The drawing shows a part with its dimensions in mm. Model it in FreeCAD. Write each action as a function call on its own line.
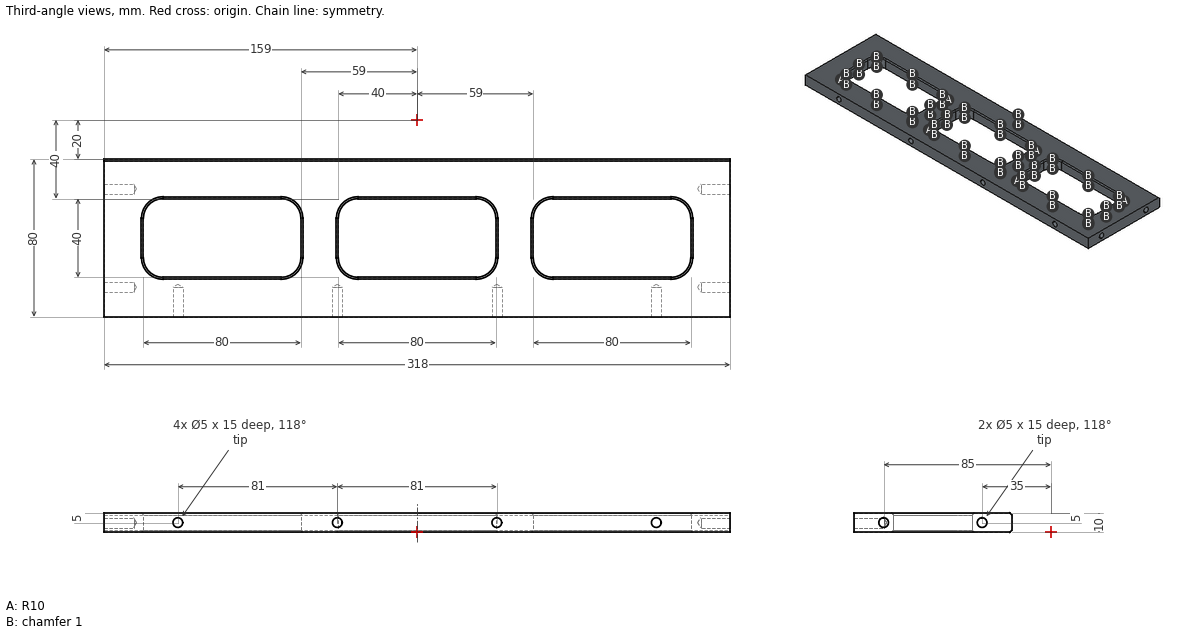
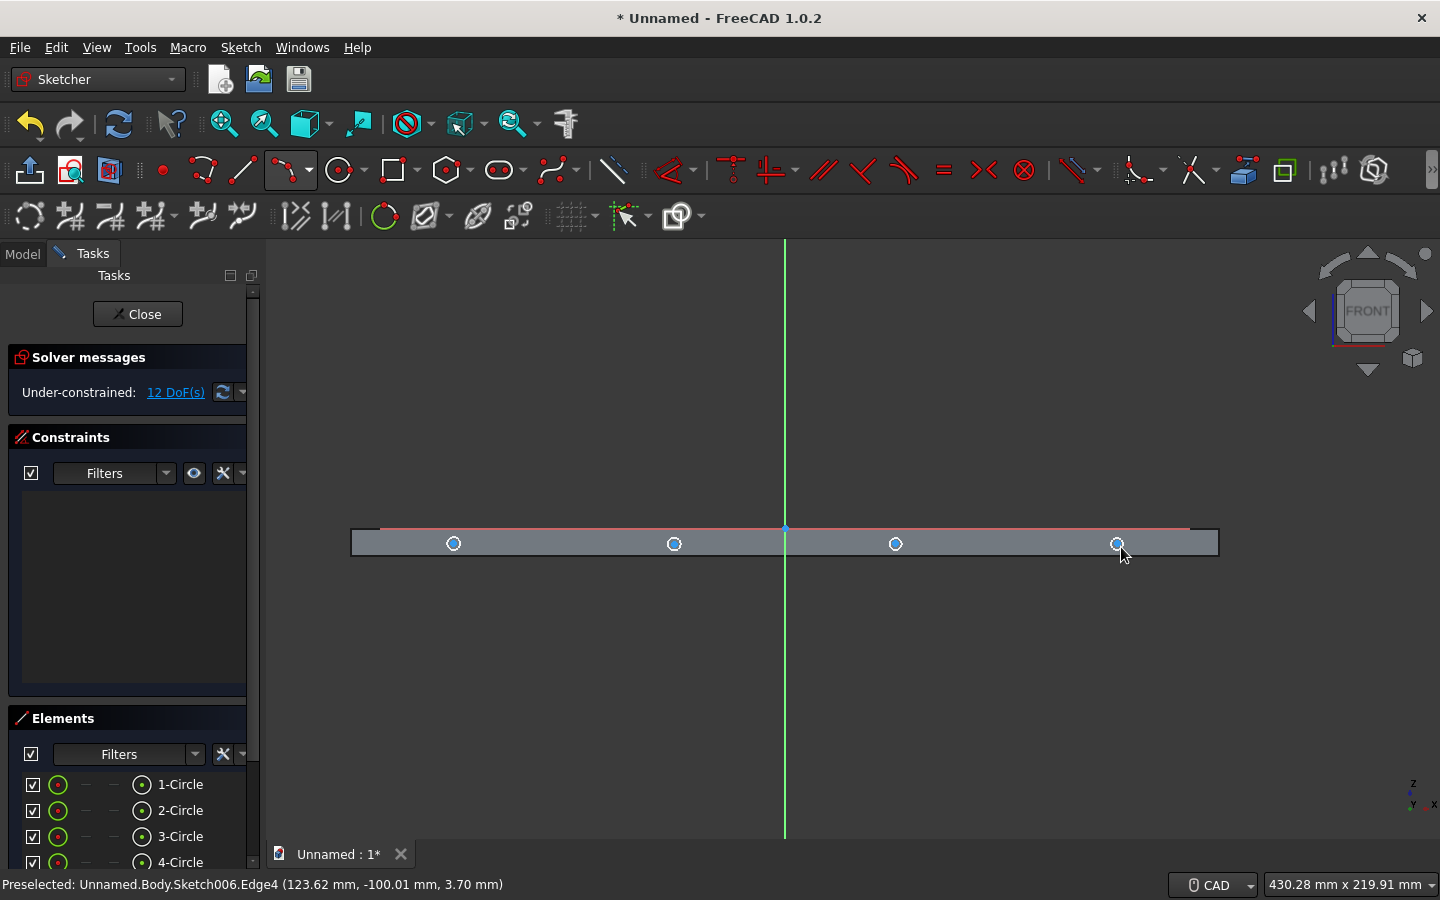
scroll(458, 539, up, 4)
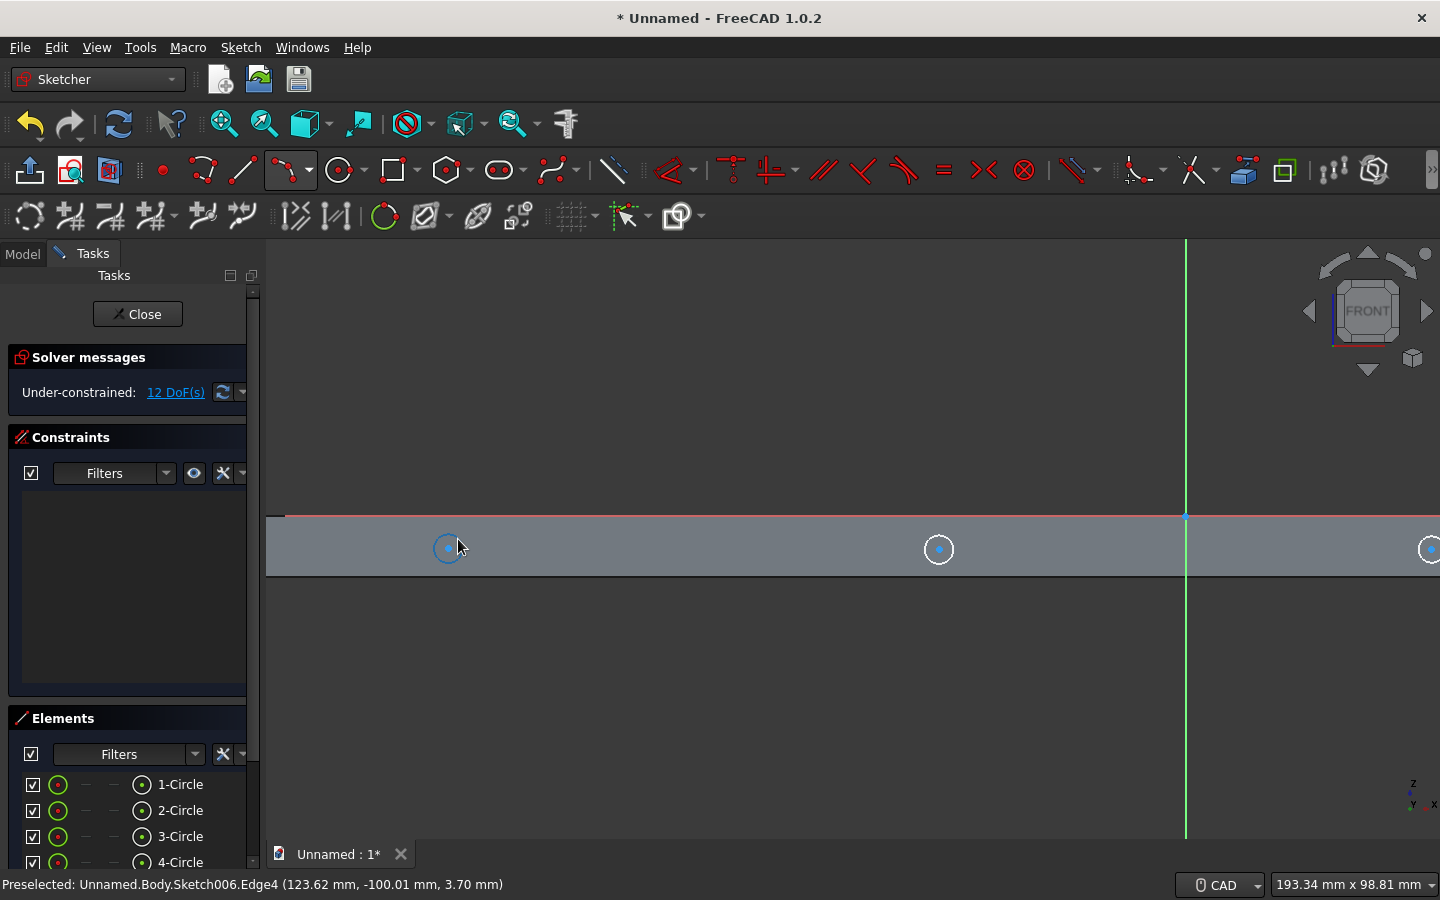
click(458, 539)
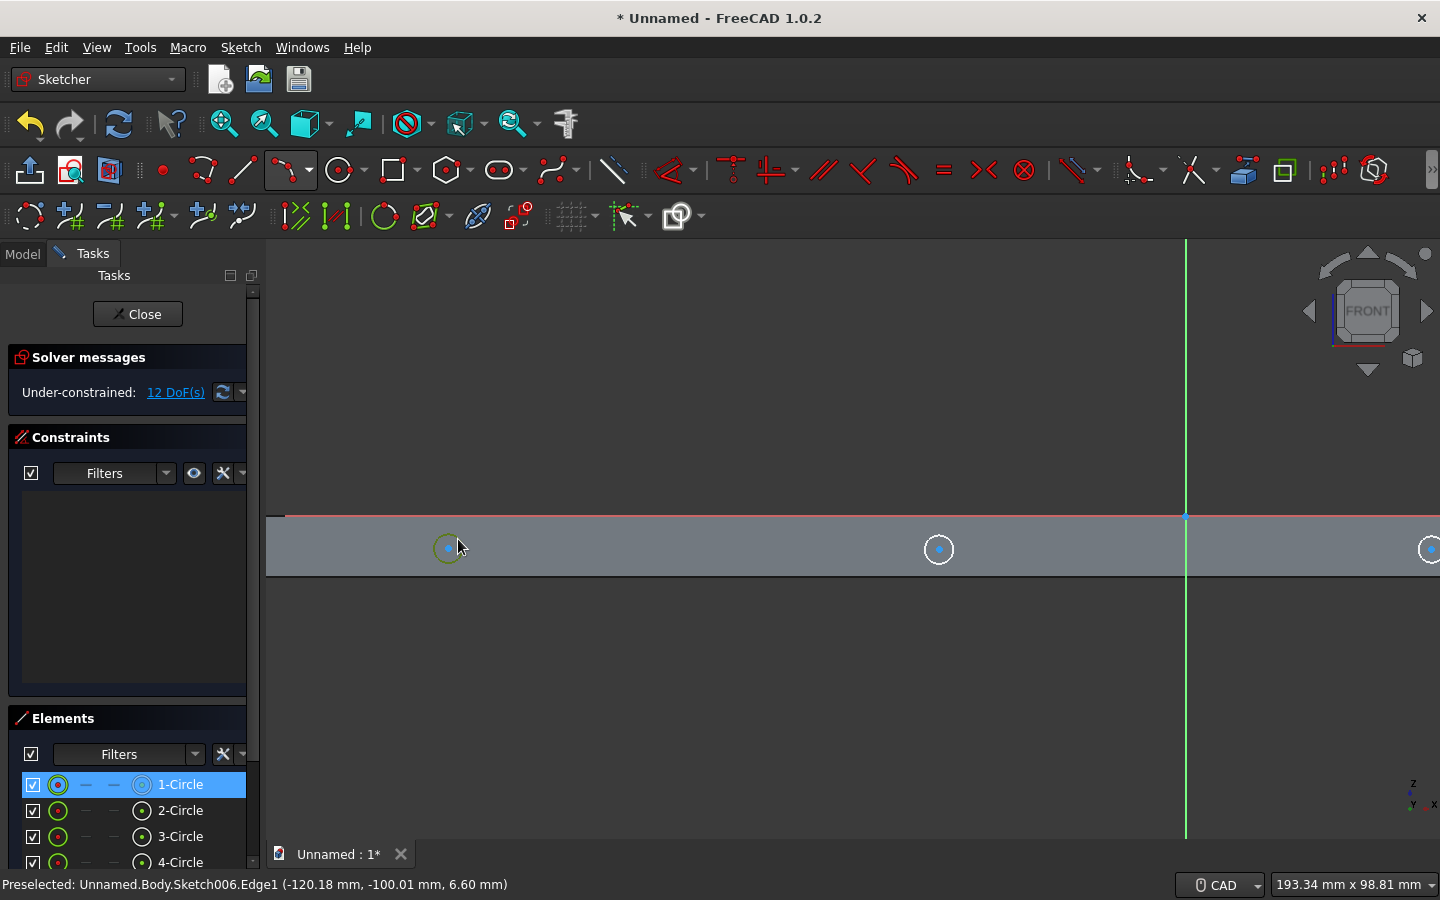
click(949, 540)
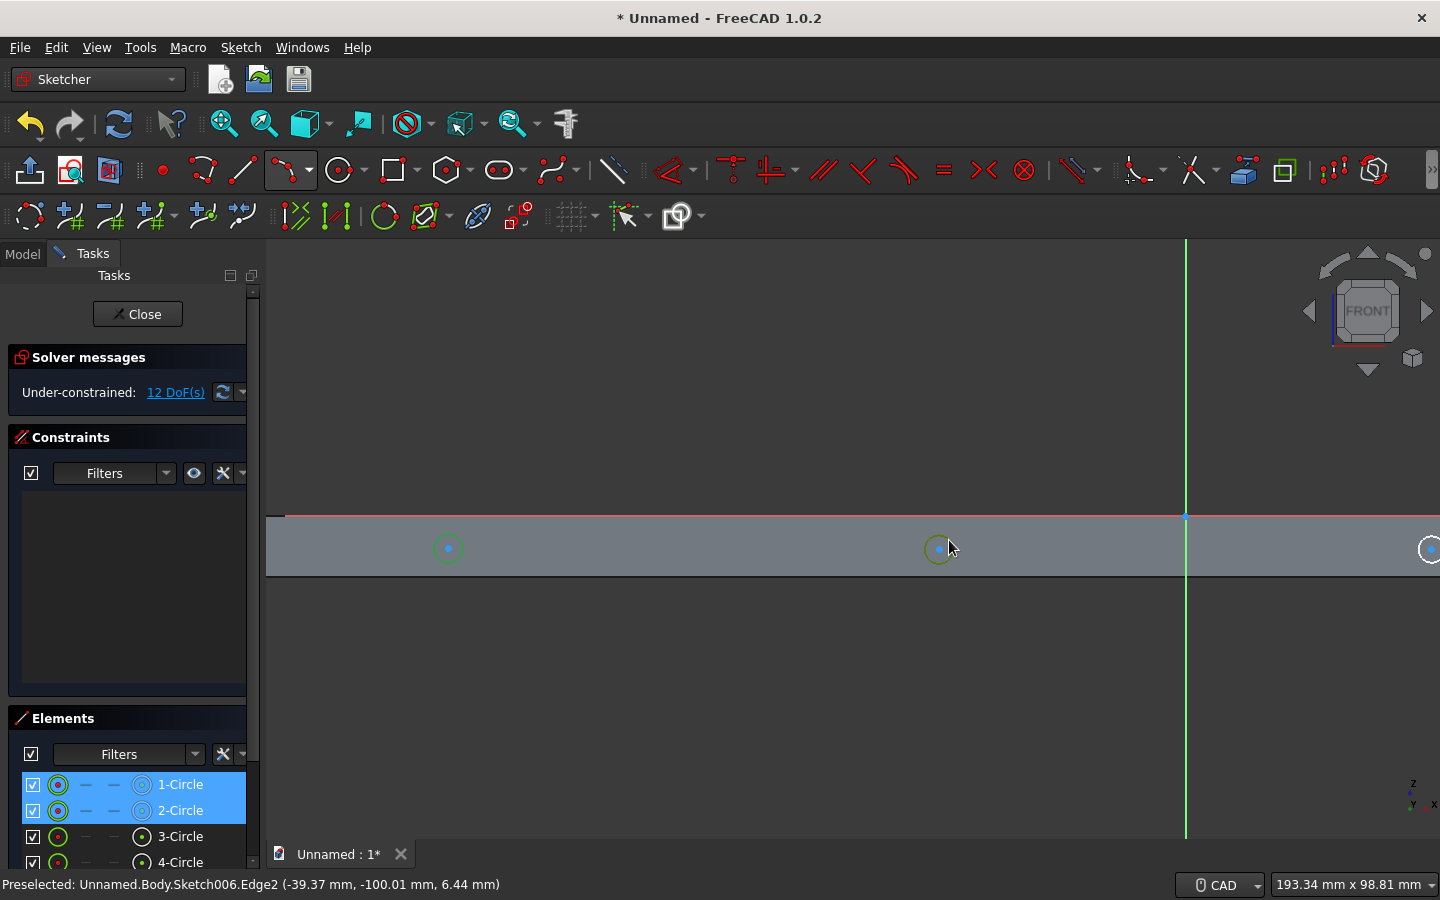
scroll(457, 539, down, 4)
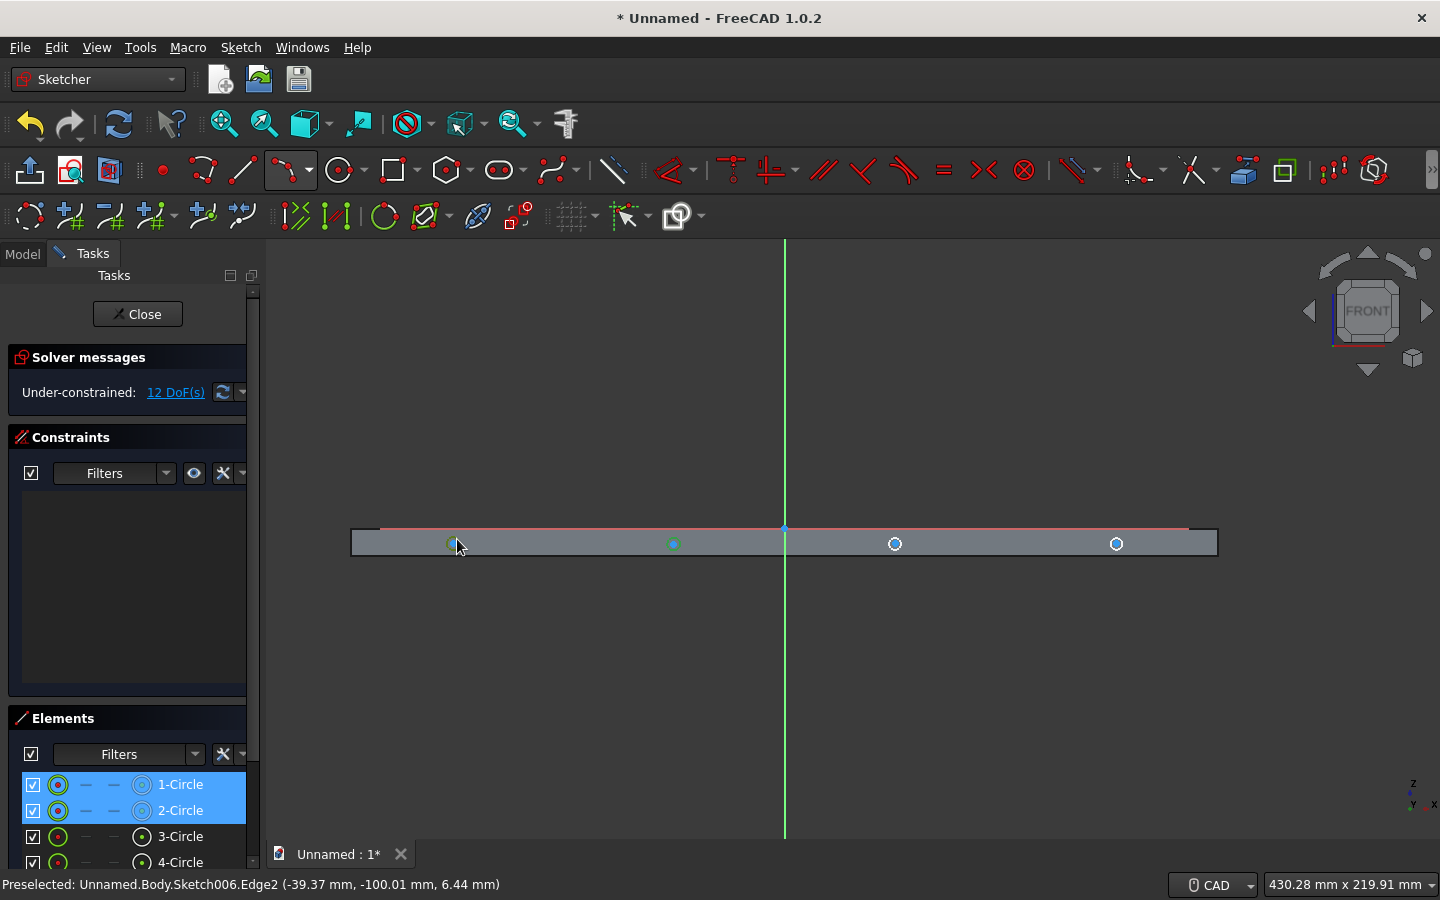
scroll(899, 540, up, 5)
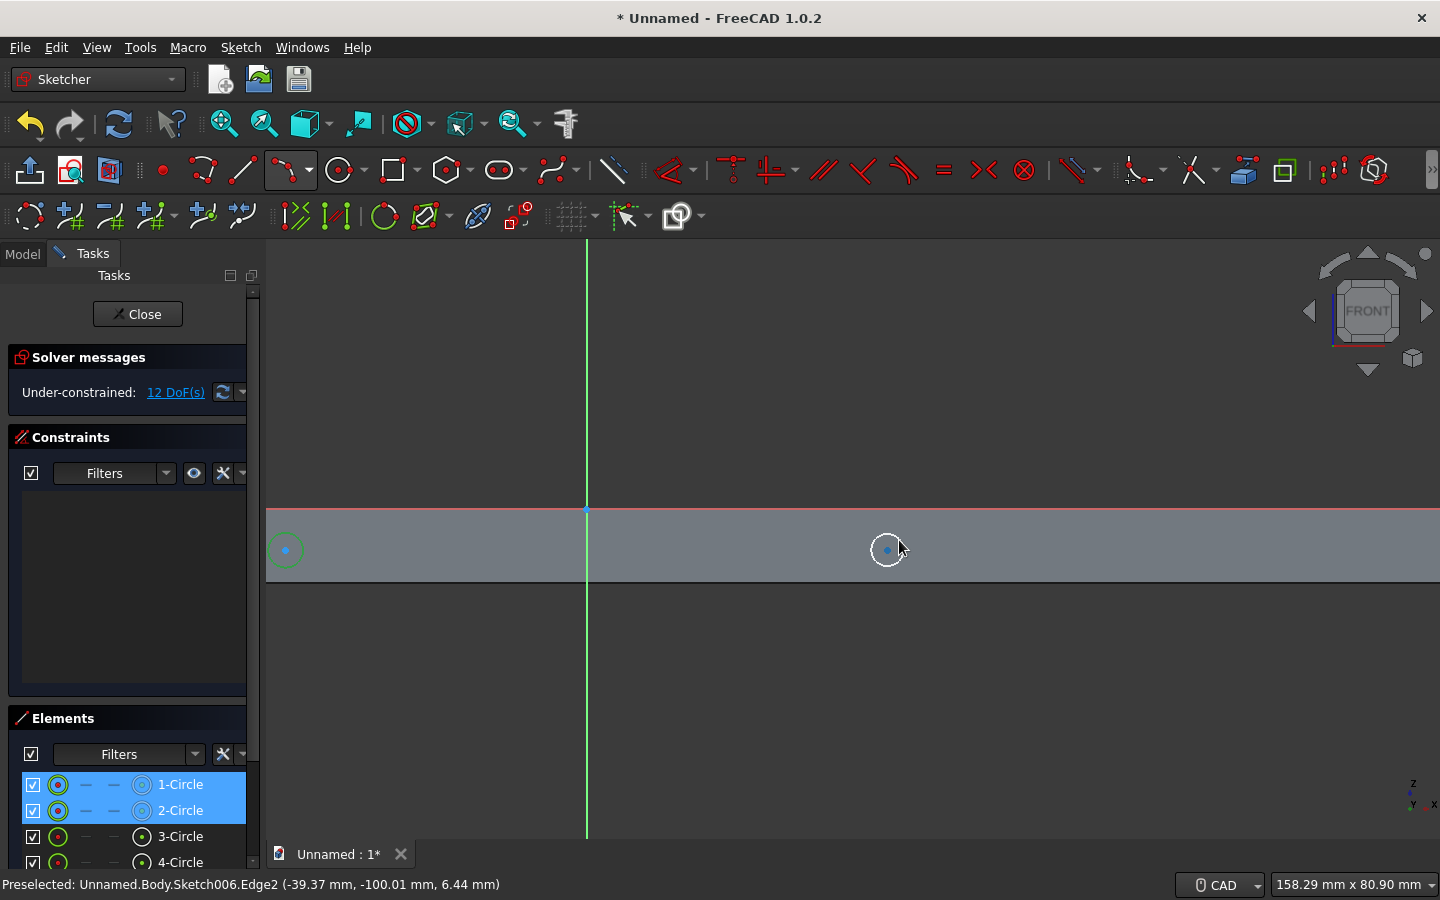
click(899, 539)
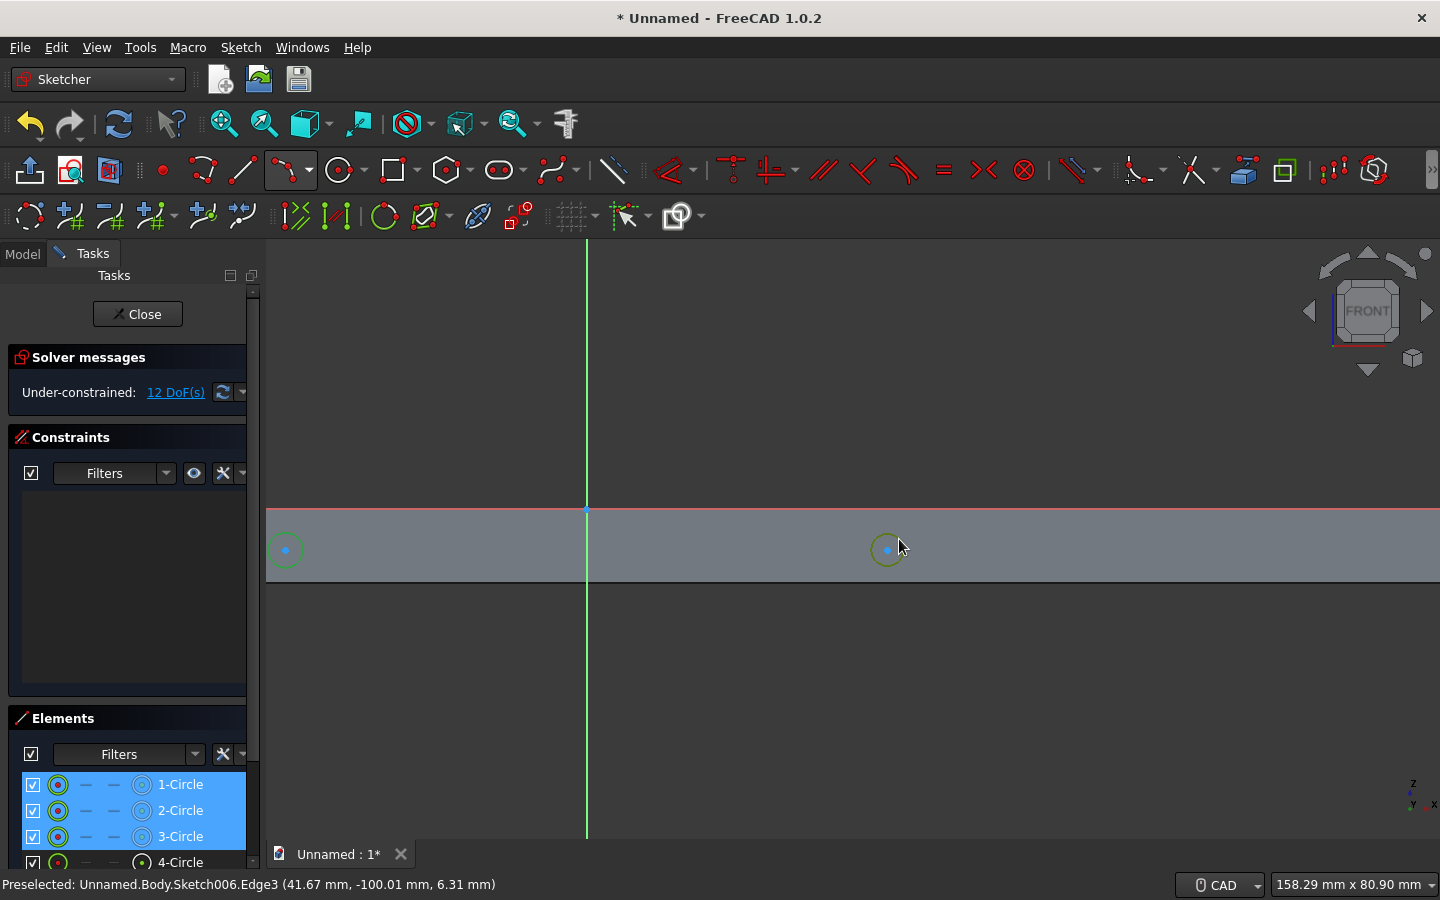
scroll(899, 540, down, 5)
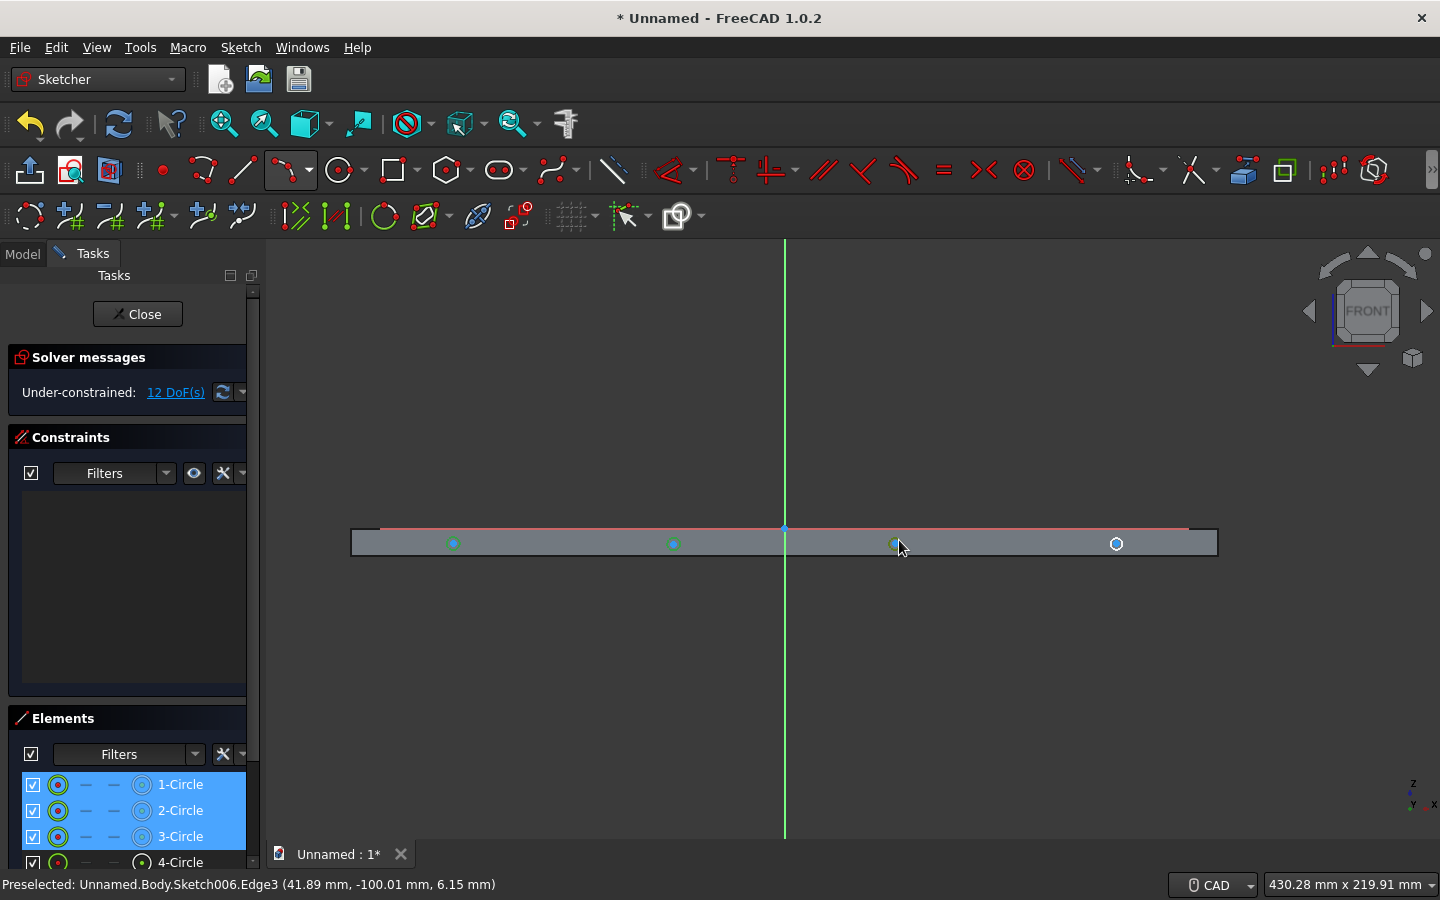
scroll(1121, 540, up, 5)